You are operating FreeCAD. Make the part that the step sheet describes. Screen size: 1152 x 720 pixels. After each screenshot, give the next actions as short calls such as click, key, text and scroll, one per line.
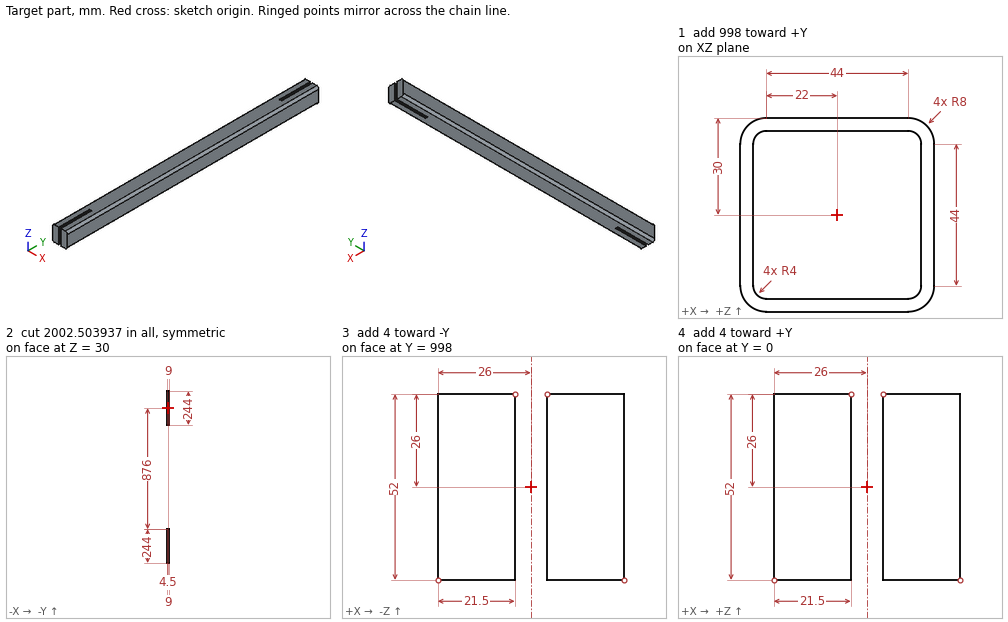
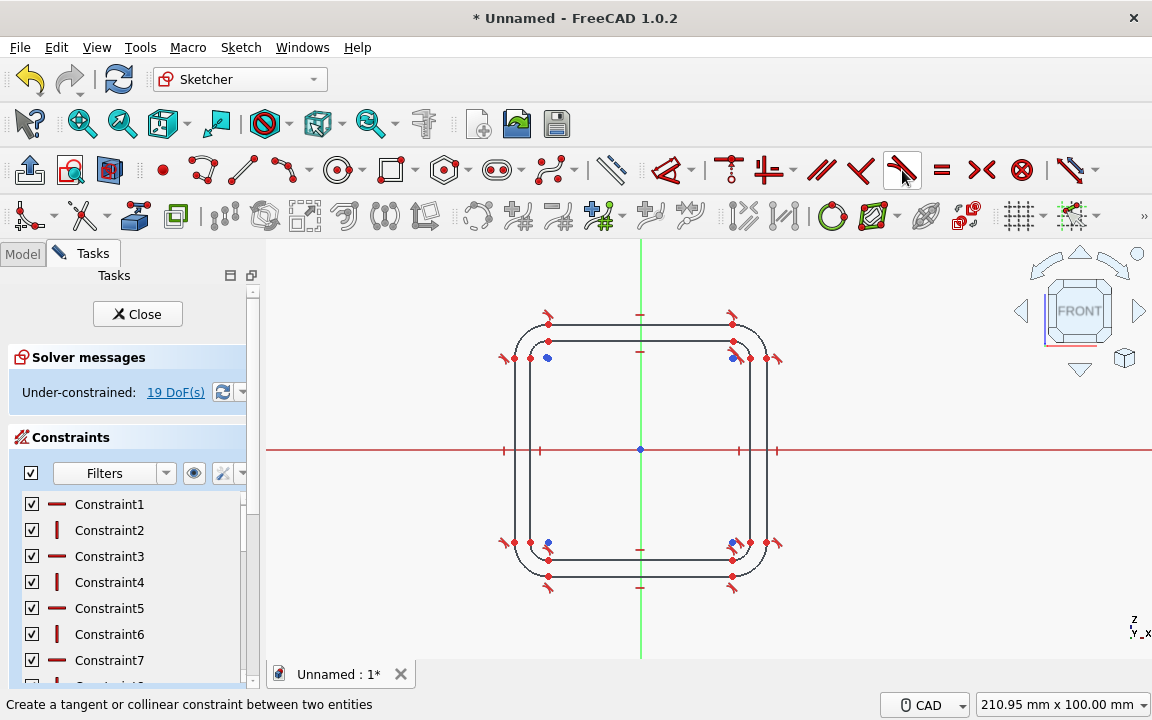
click(678, 341)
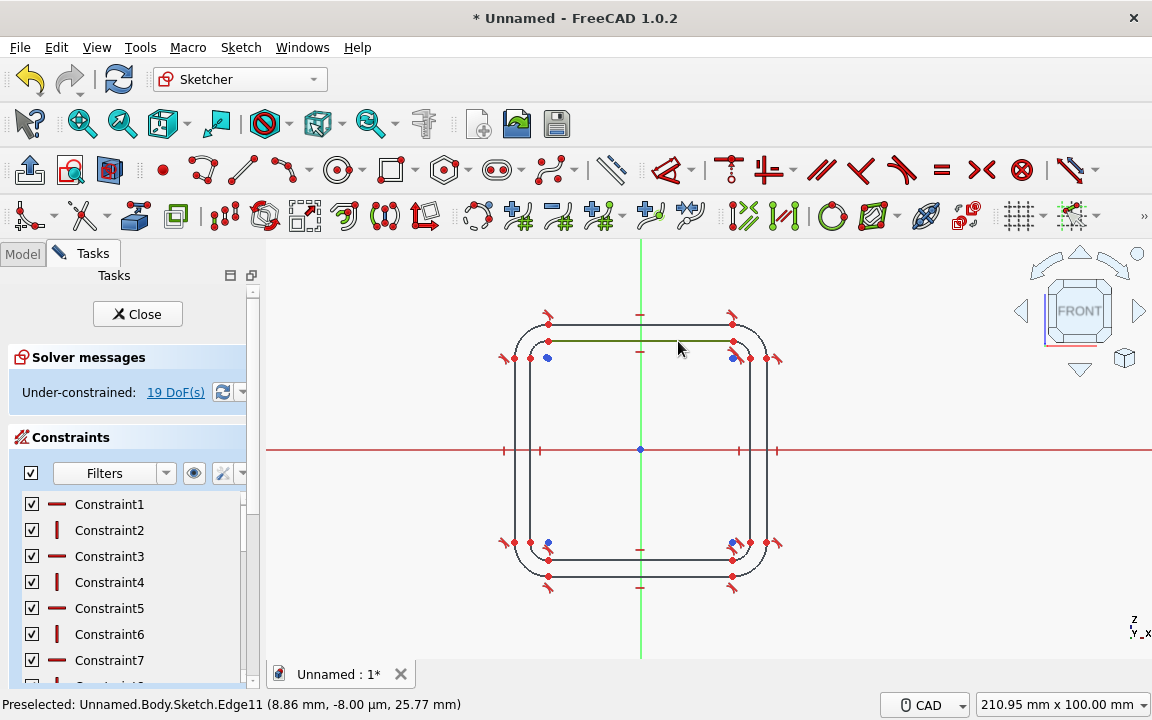
click(535, 346)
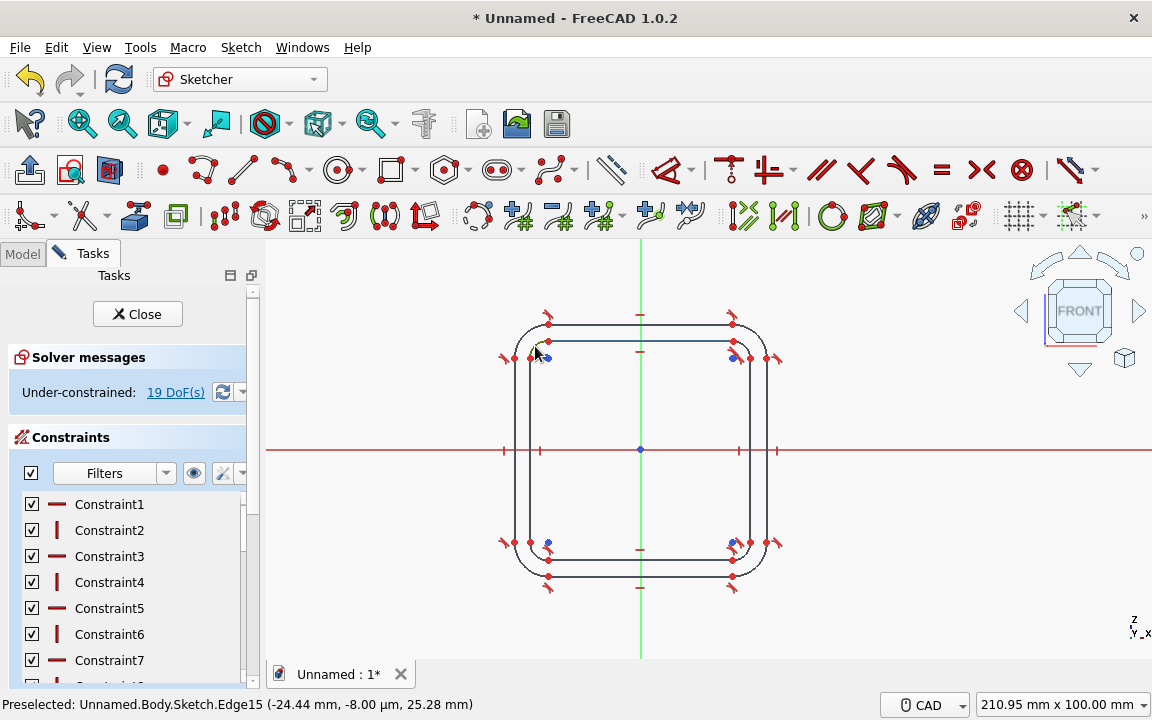
click(902, 170)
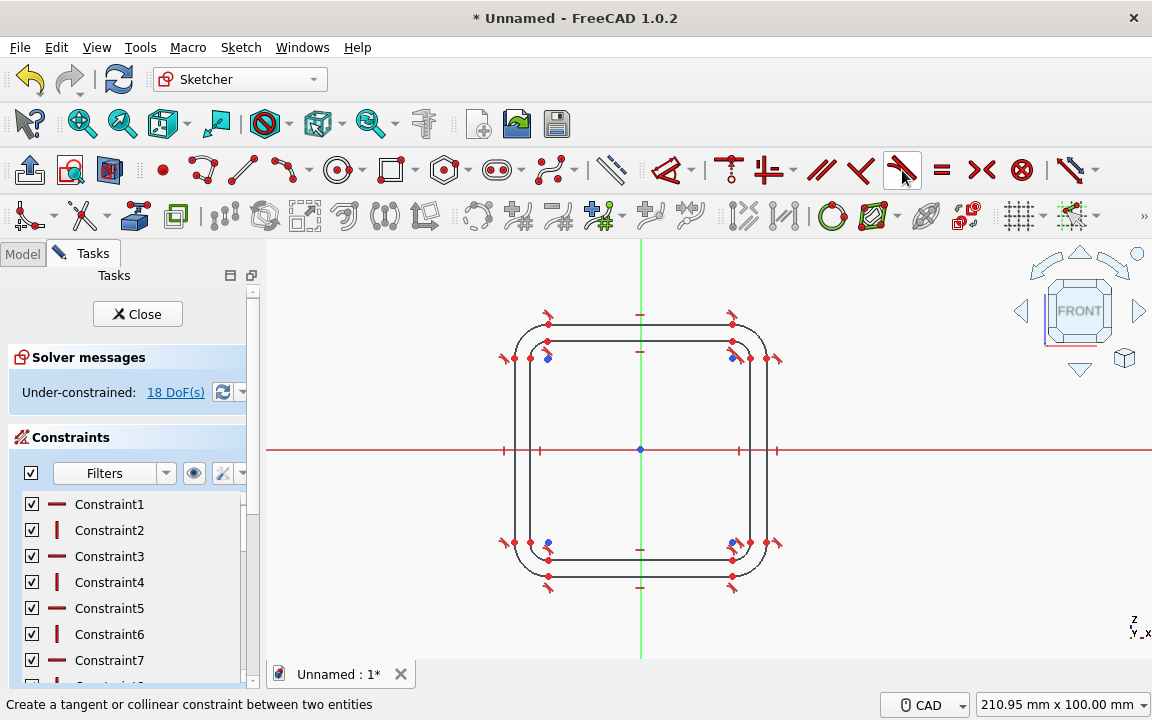
click(530, 414)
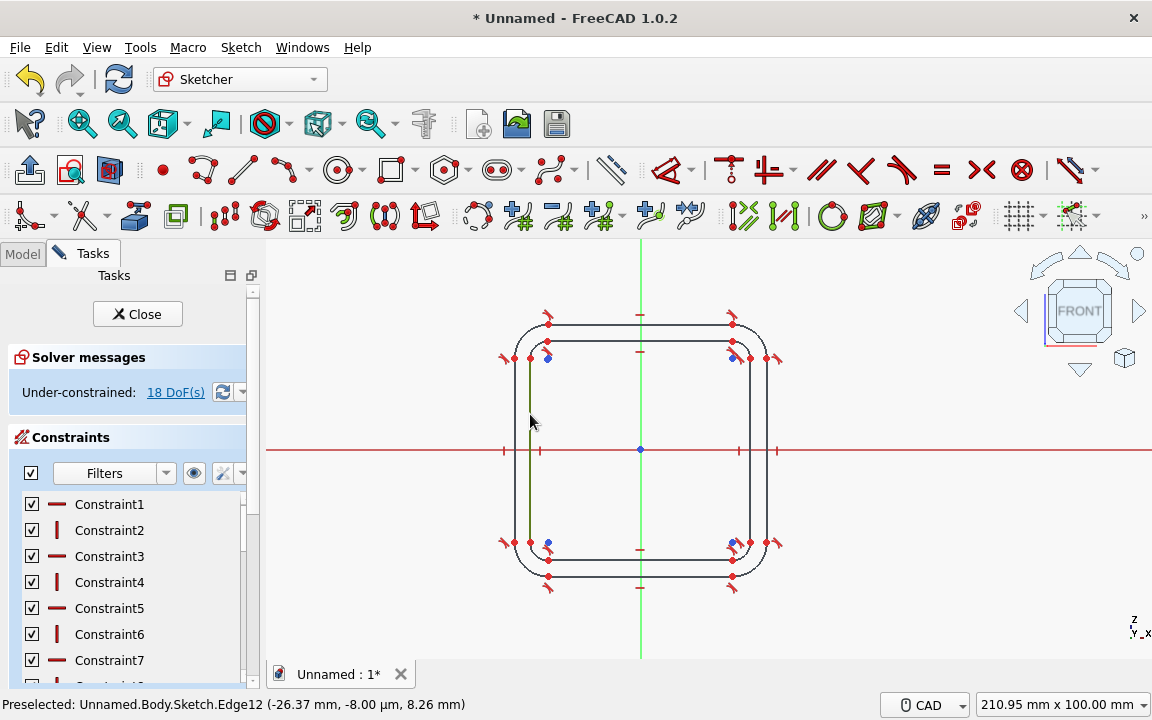
click(536, 346)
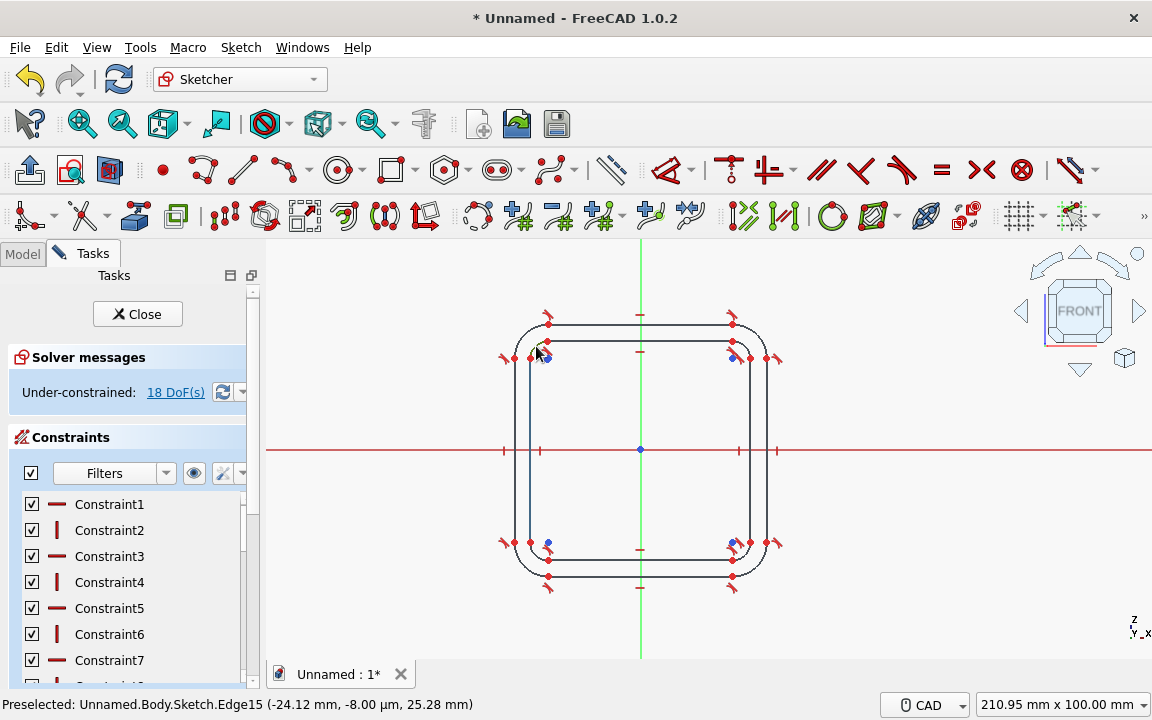
click(902, 170)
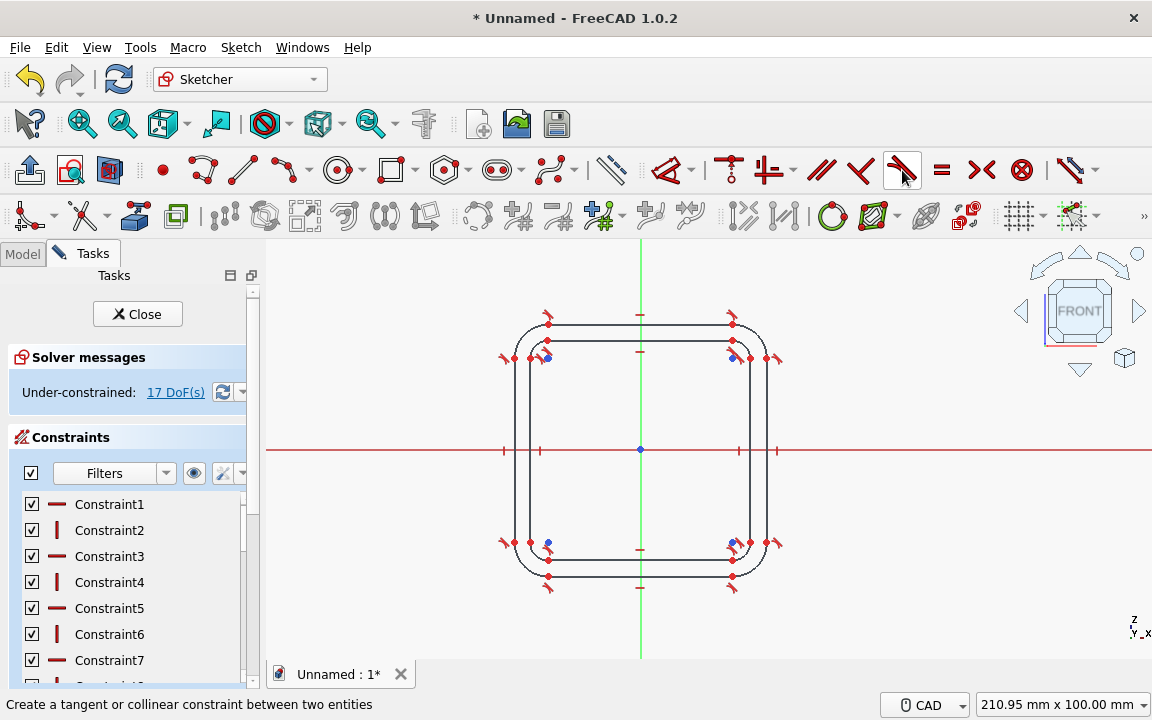
click(530, 414)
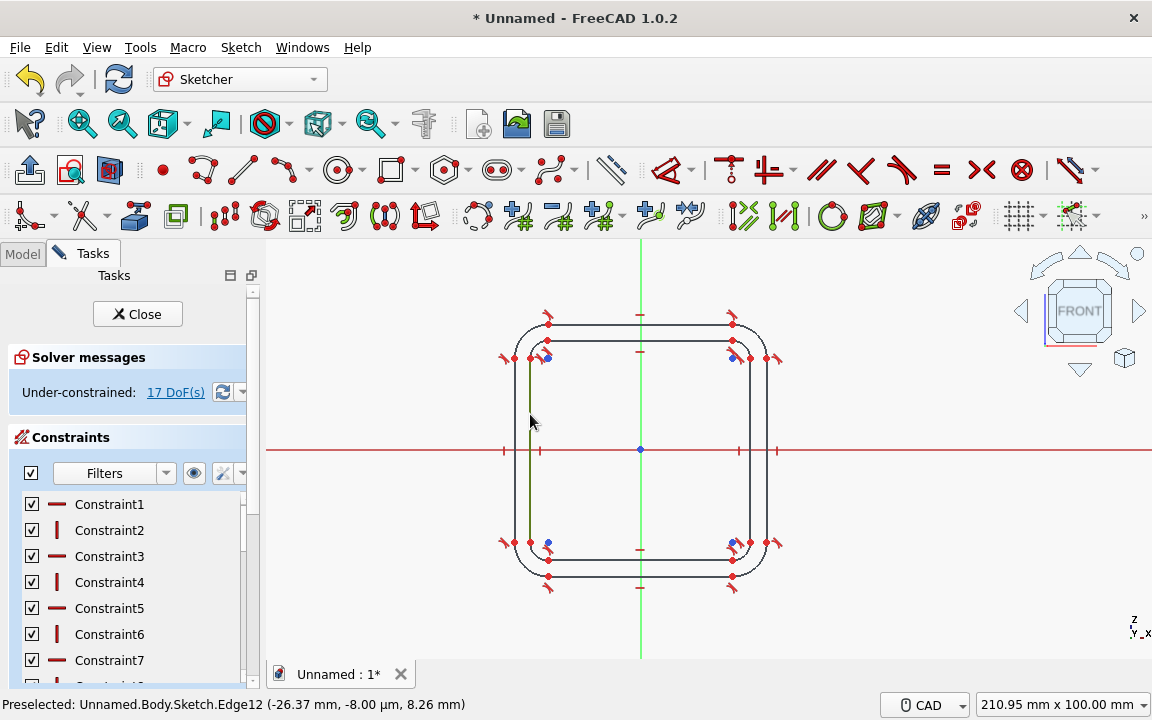
click(535, 555)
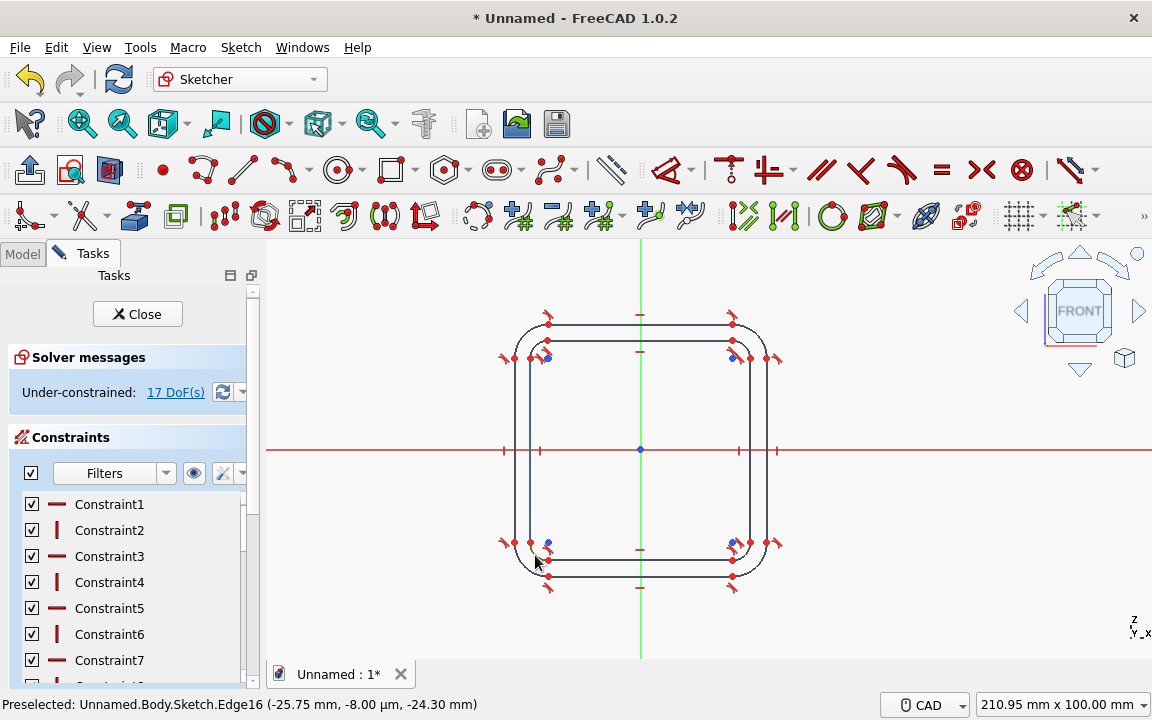
key(t)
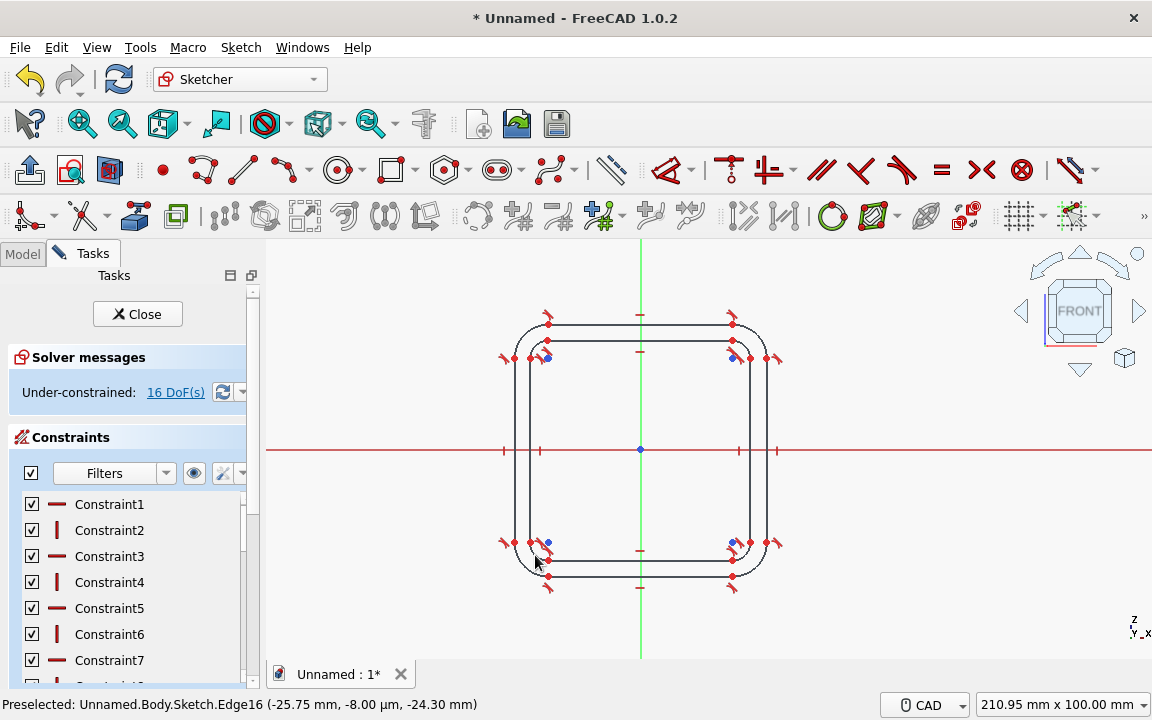
click(748, 573)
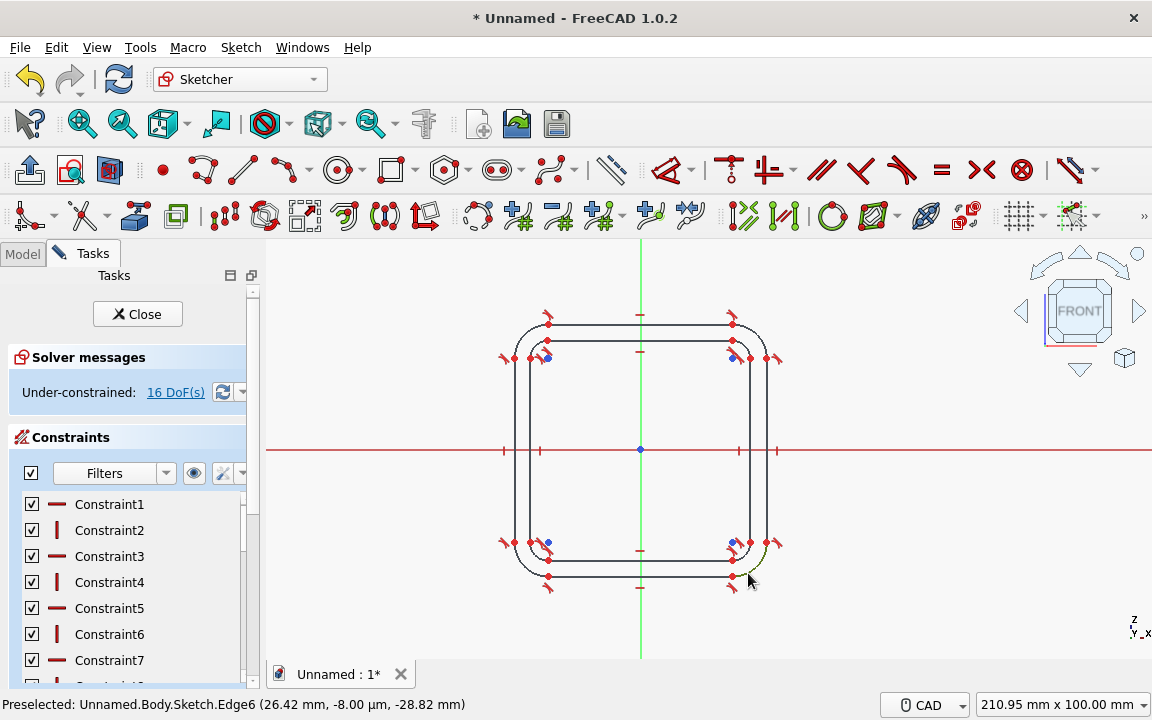
click(745, 555)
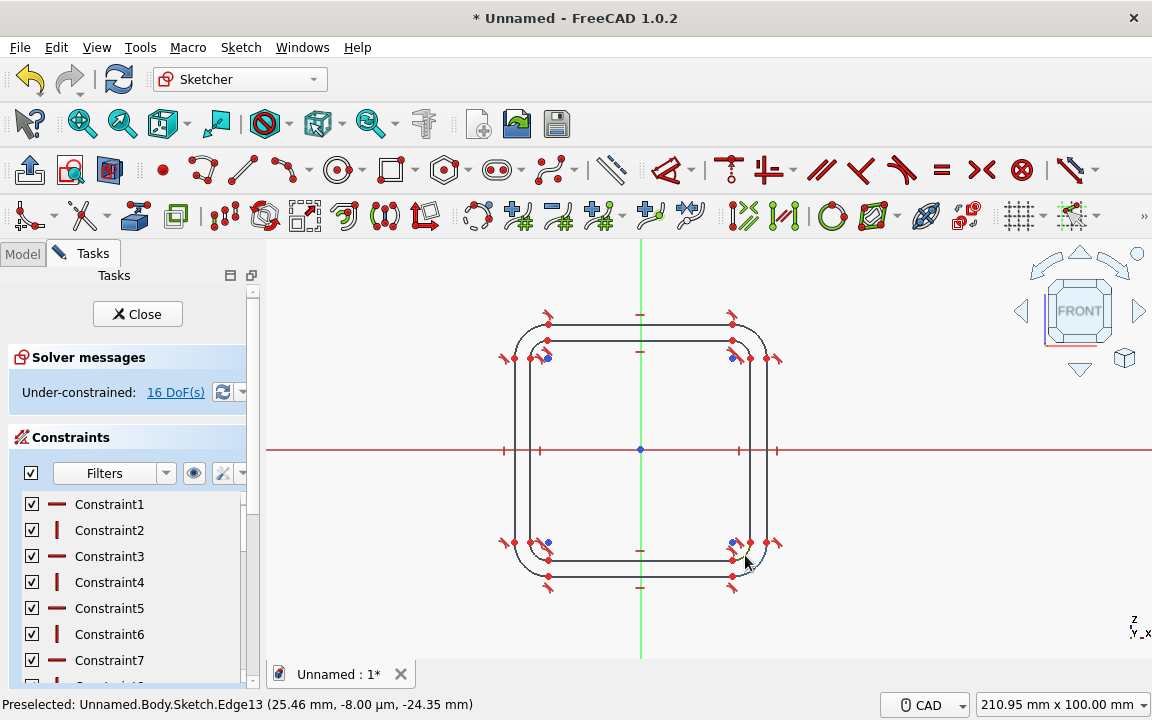
click(730, 170)